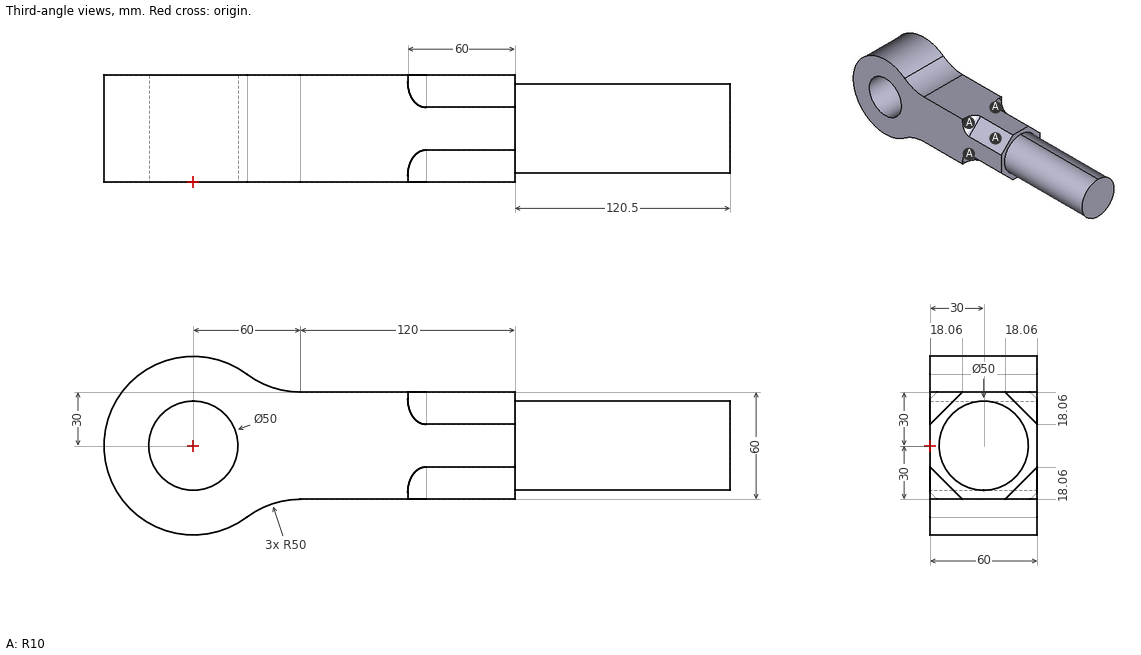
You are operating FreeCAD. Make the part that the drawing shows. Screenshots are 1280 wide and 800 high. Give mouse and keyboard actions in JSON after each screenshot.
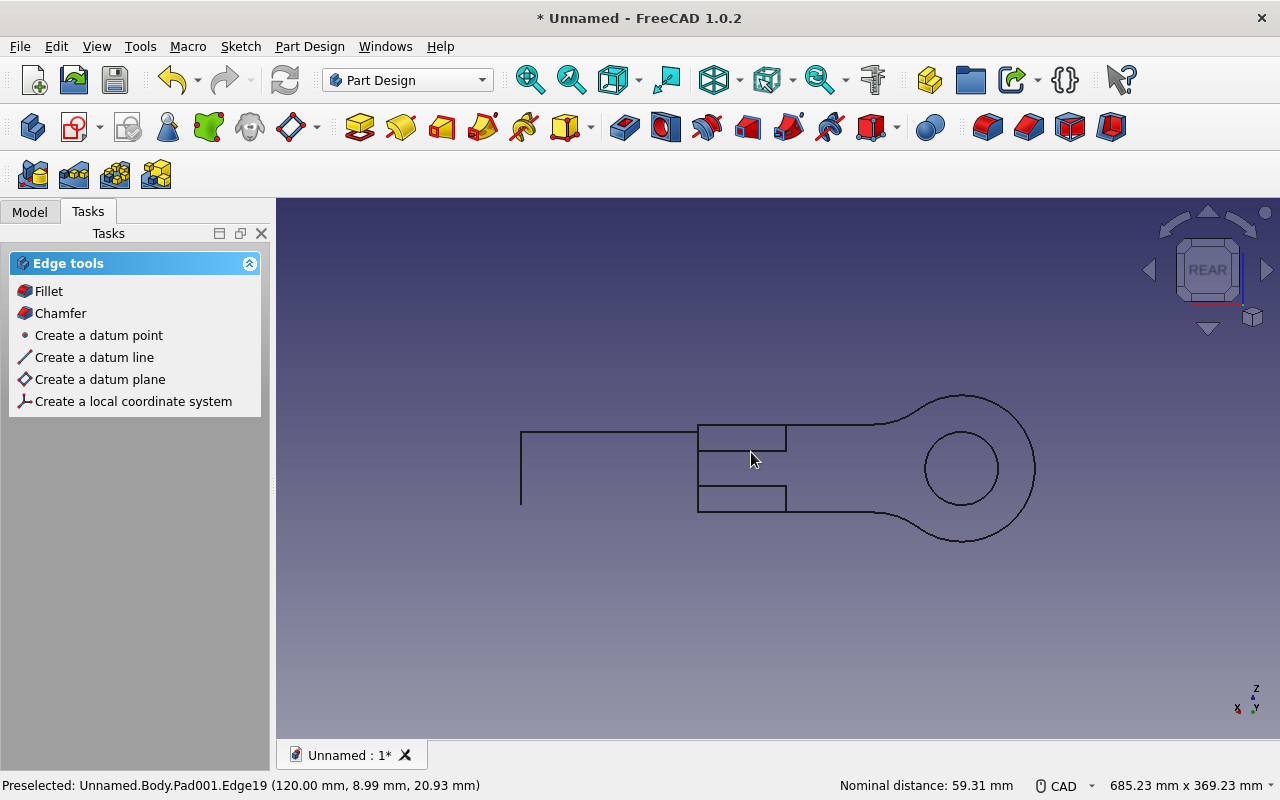
{"action": "key", "text": "6"}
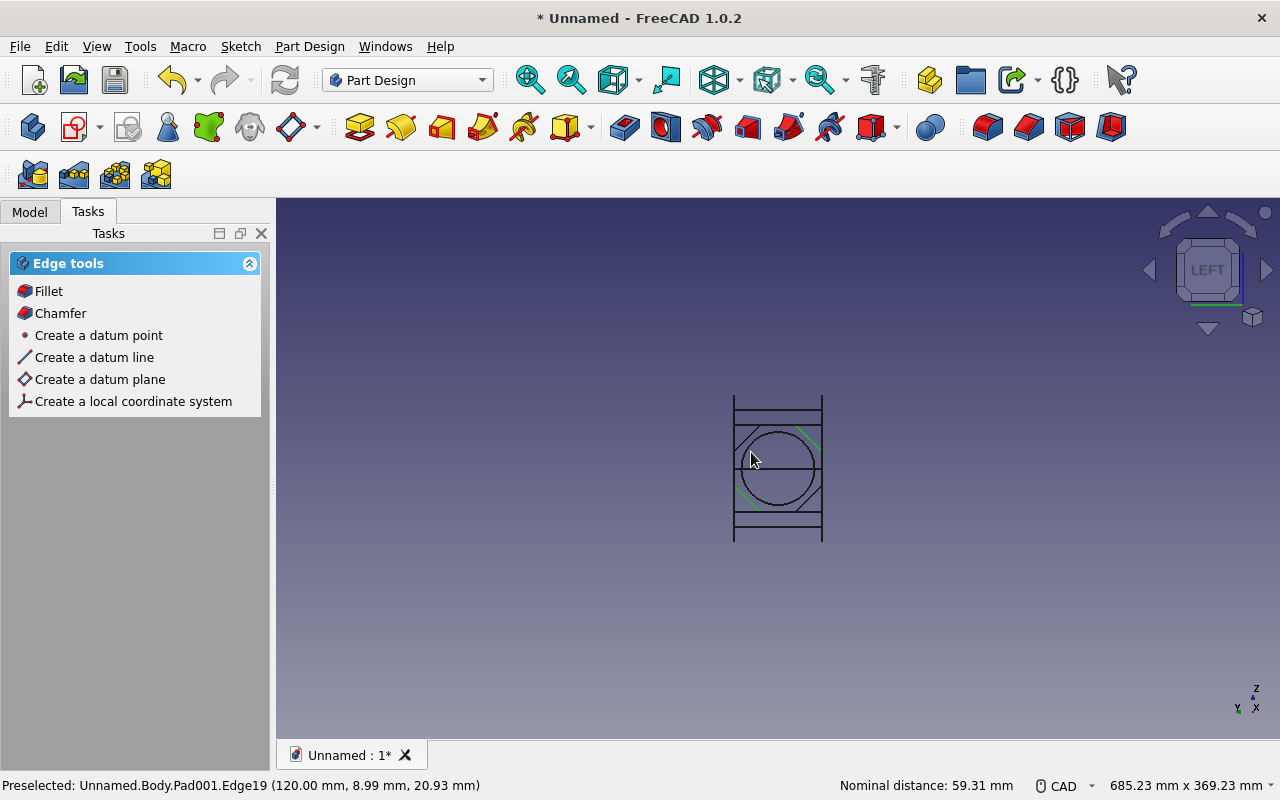
{"action": "key", "text": "v f"}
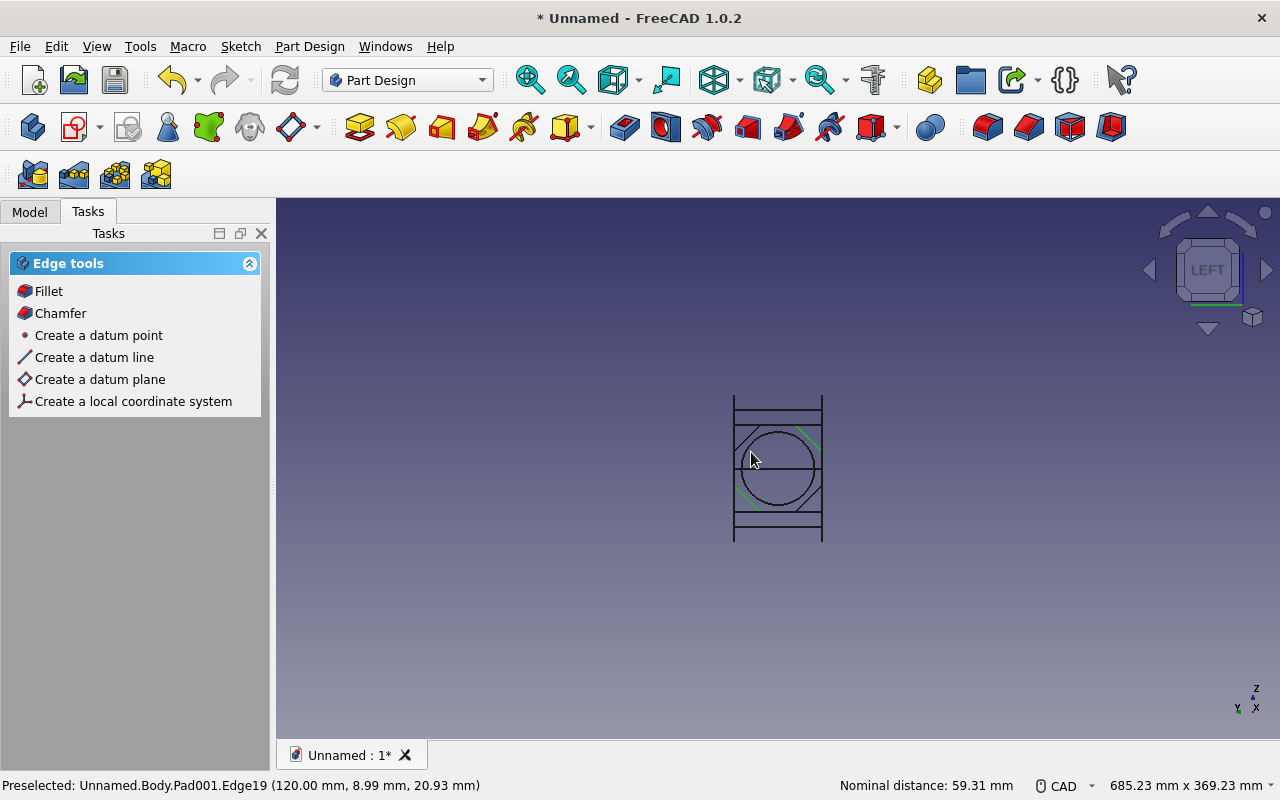
{"action": "left_click", "coordinate": [809, 498], "text": "ctrl"}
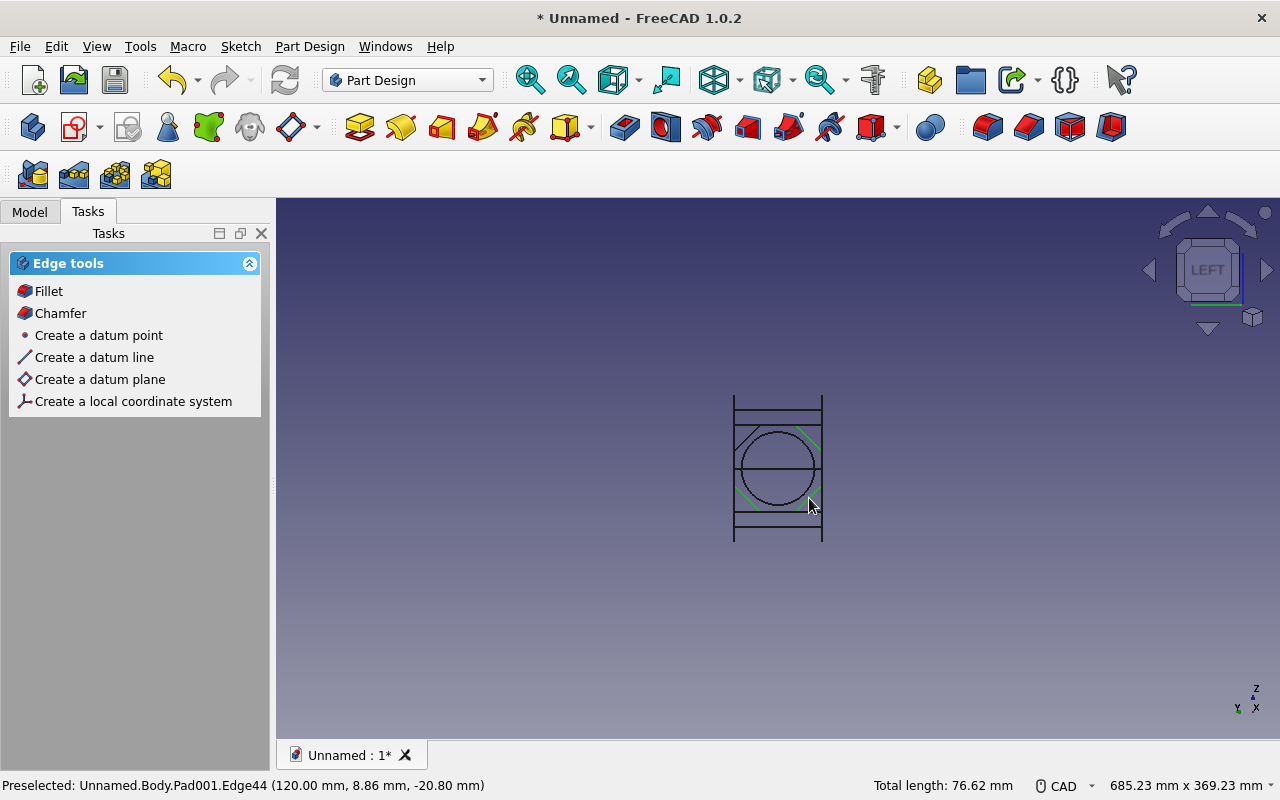
{"action": "left_click", "coordinate": [747, 437], "text": "ctrl"}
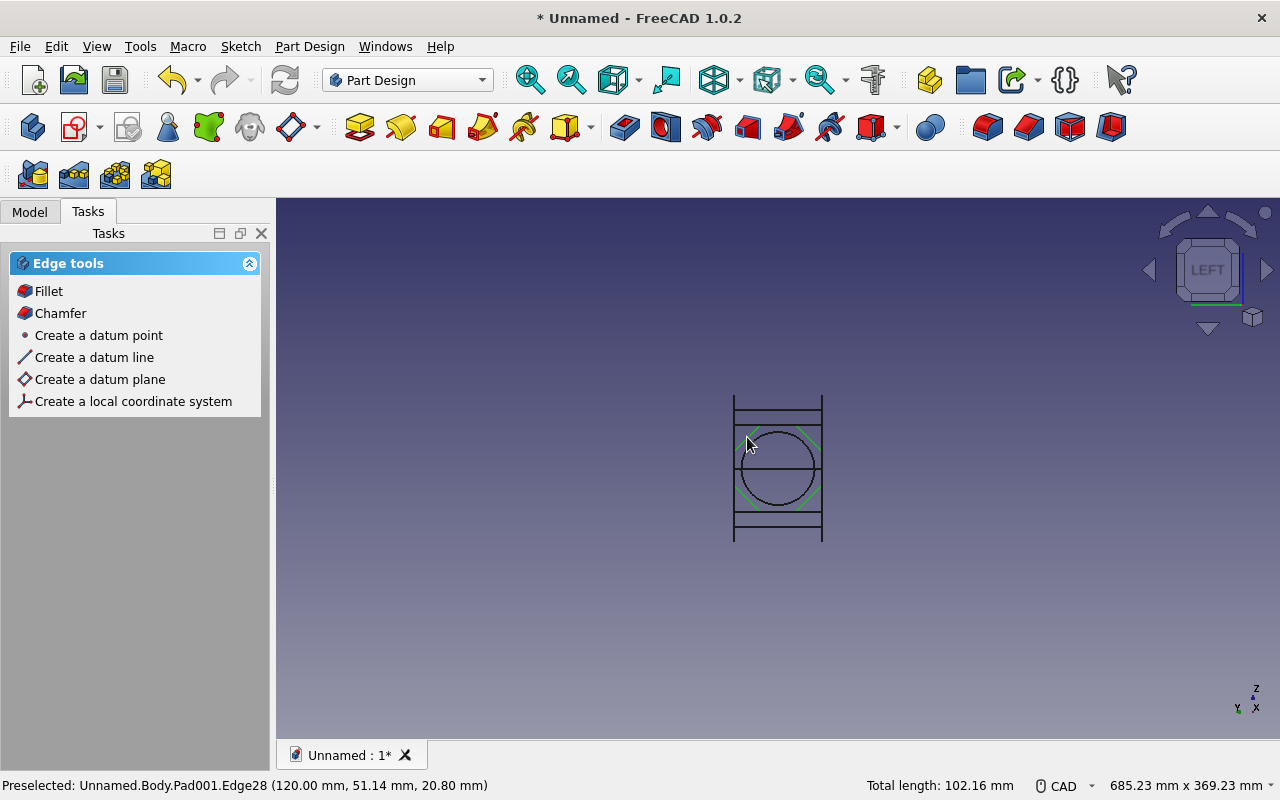
{"action": "key", "text": "v 1"}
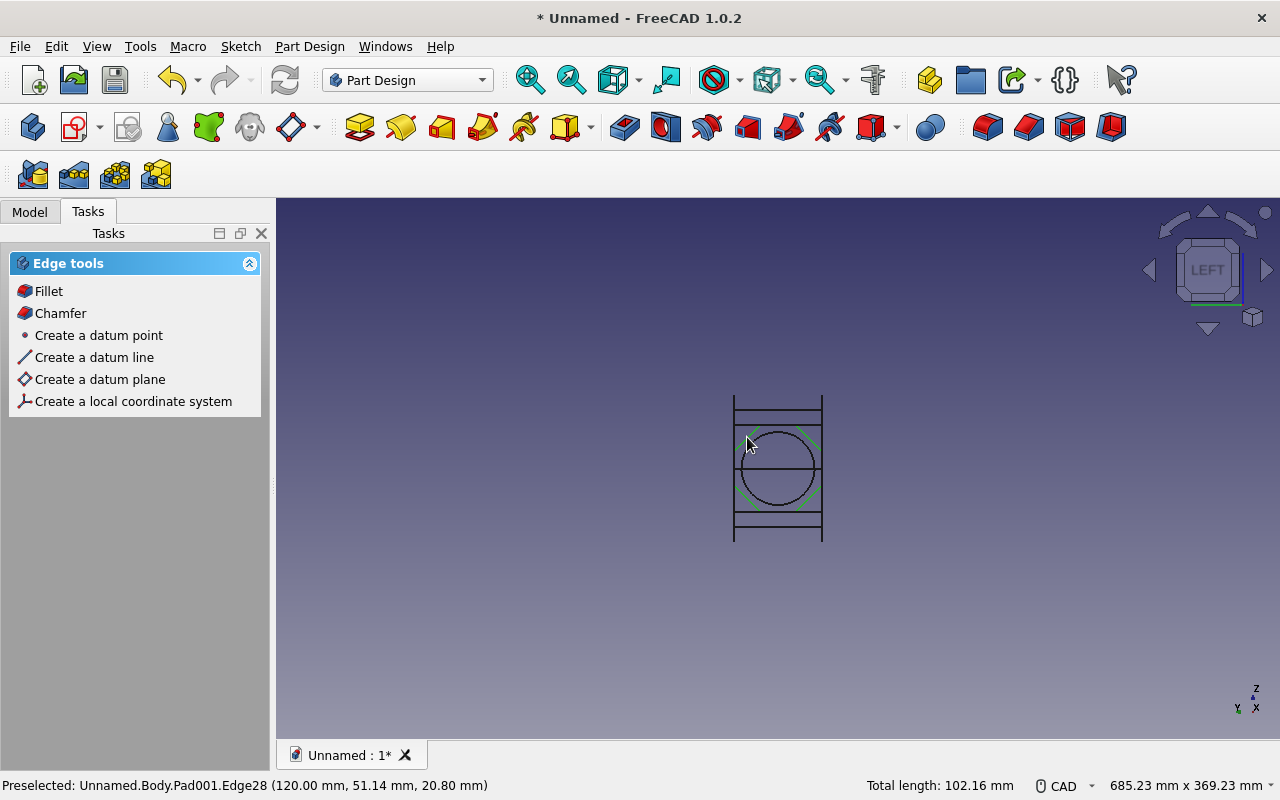
{"action": "left_click", "coordinate": [988, 128]}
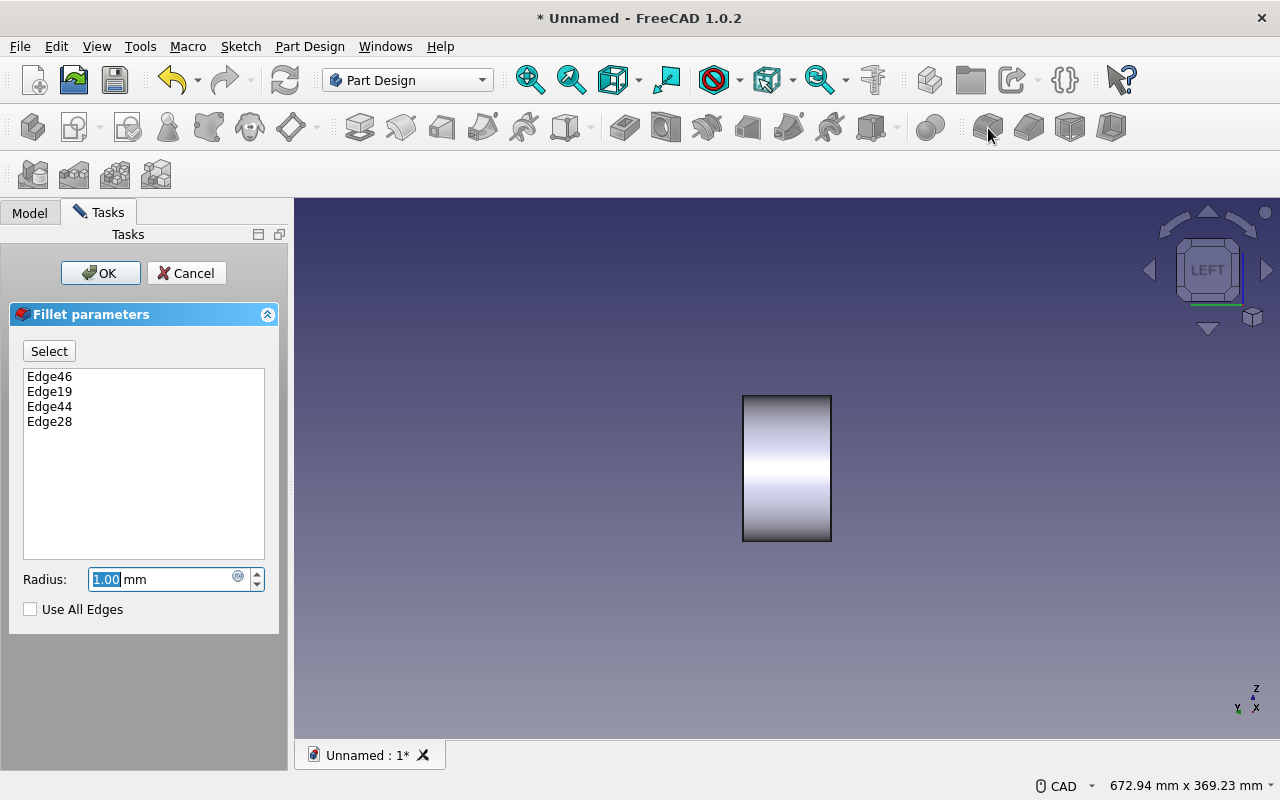
{"action": "type", "text": "10"}
{"action": "key", "text": "Tab"}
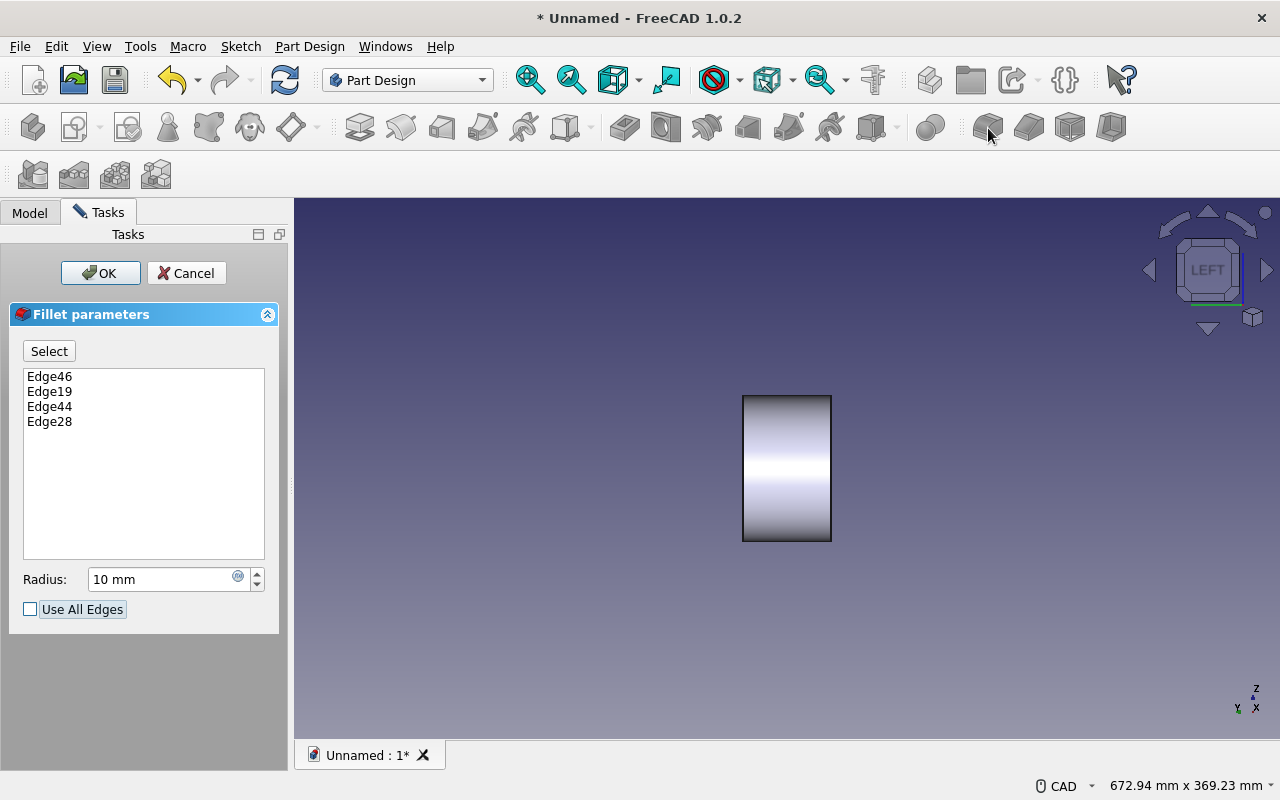
{"action": "left_click", "coordinate": [101, 273]}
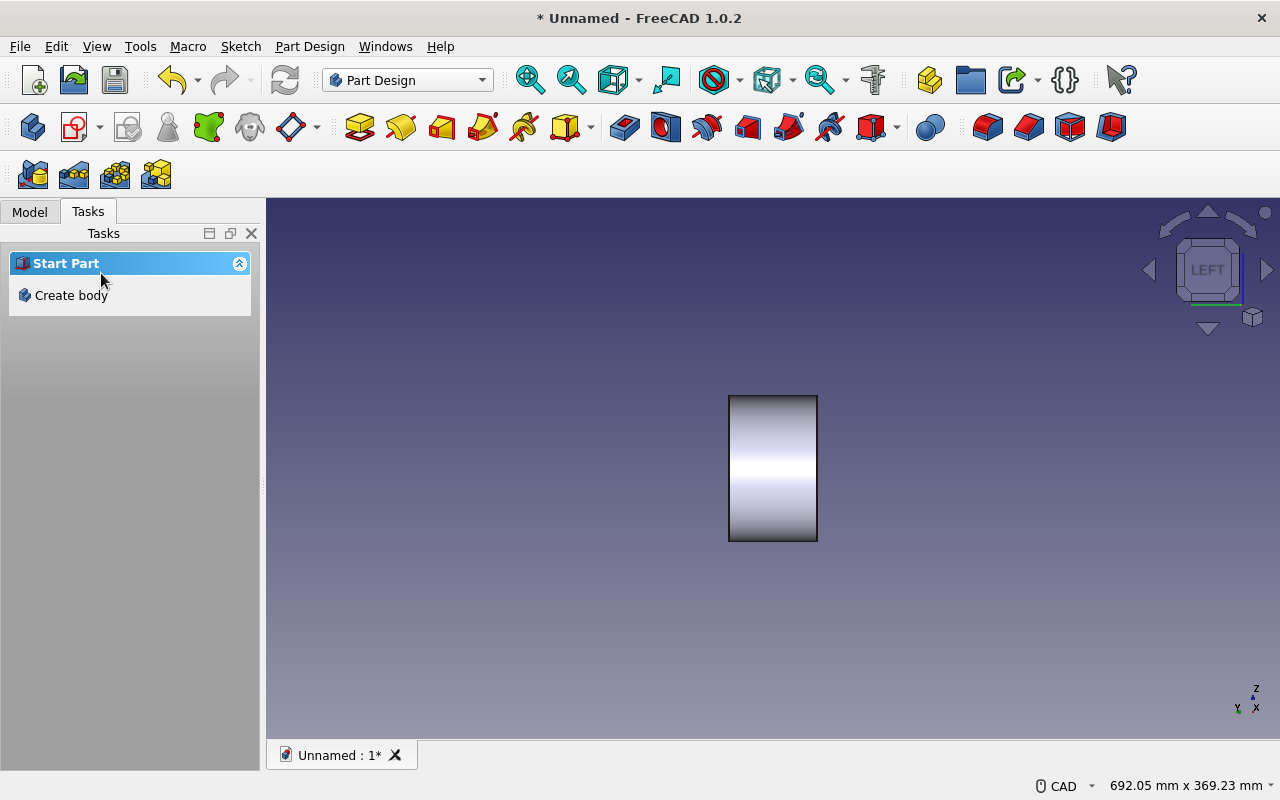
{"action": "key", "text": "0"}